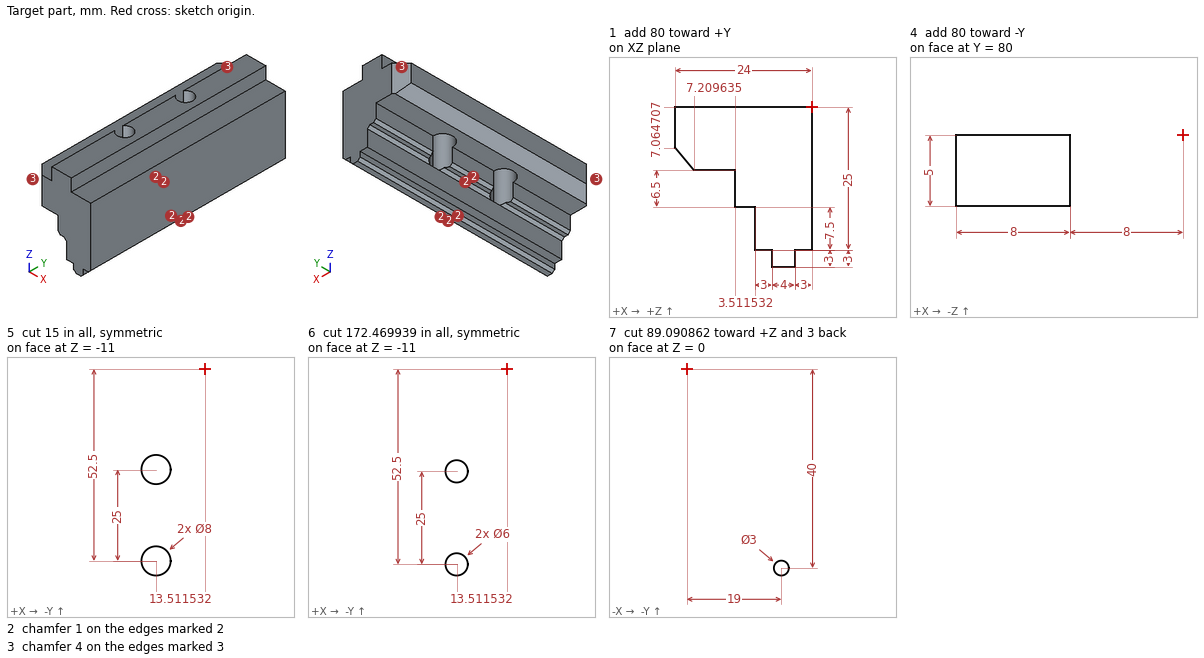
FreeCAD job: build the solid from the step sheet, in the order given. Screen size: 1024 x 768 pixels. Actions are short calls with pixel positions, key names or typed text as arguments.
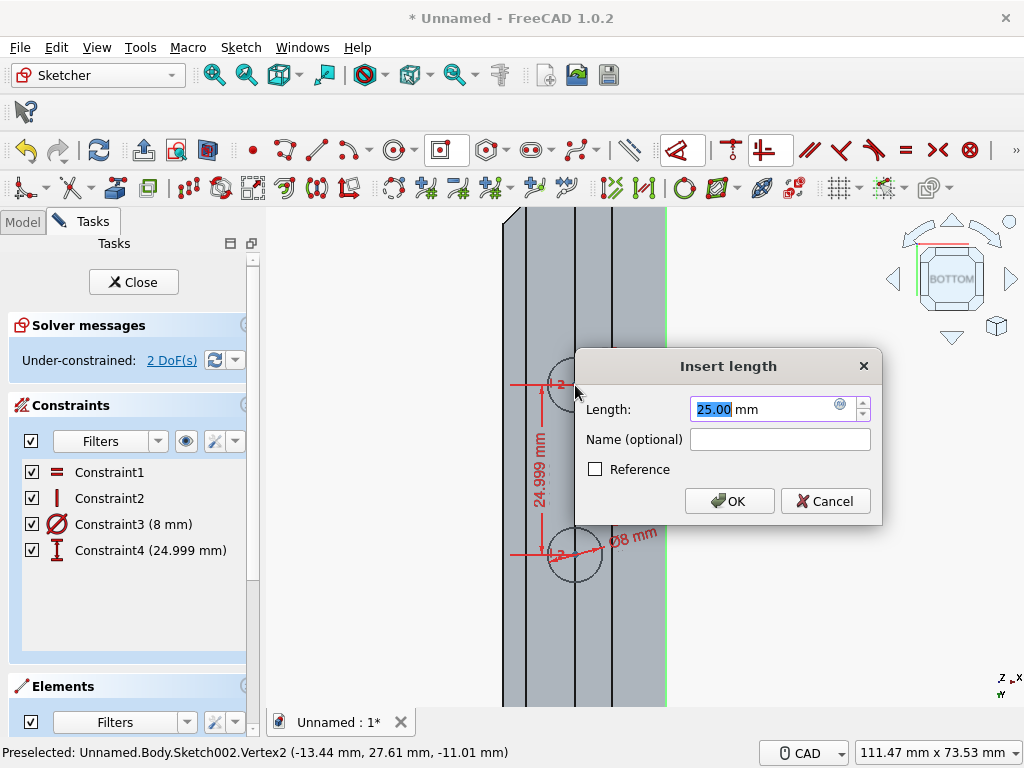
text(25)
key(Return)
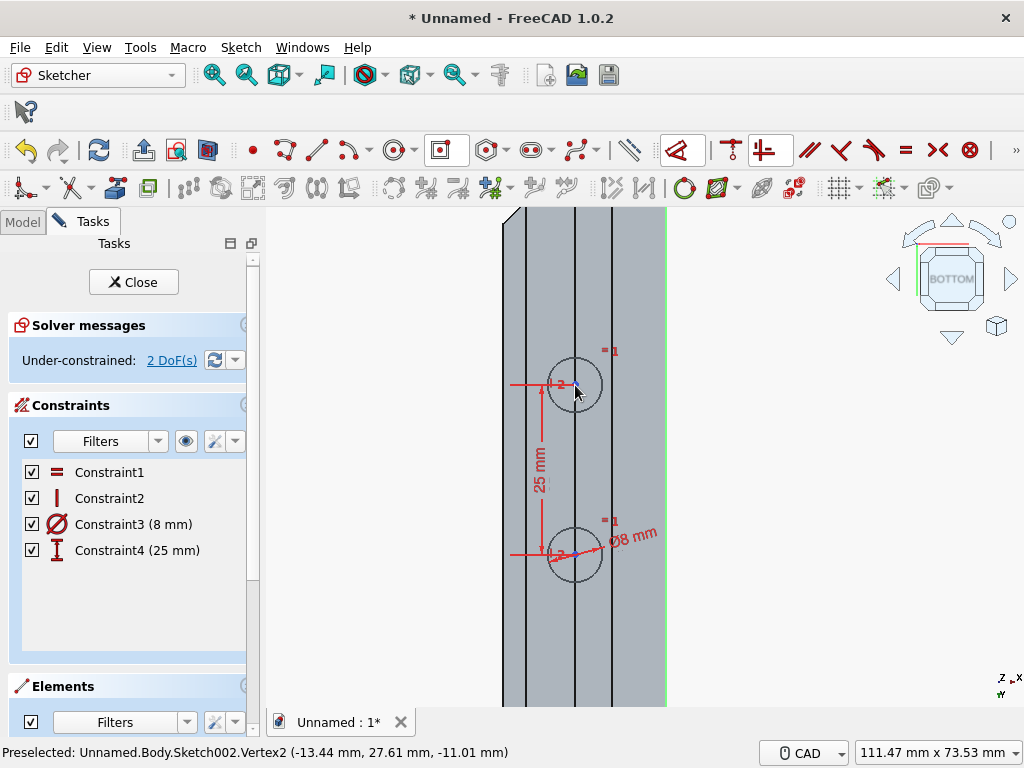
click(575, 555)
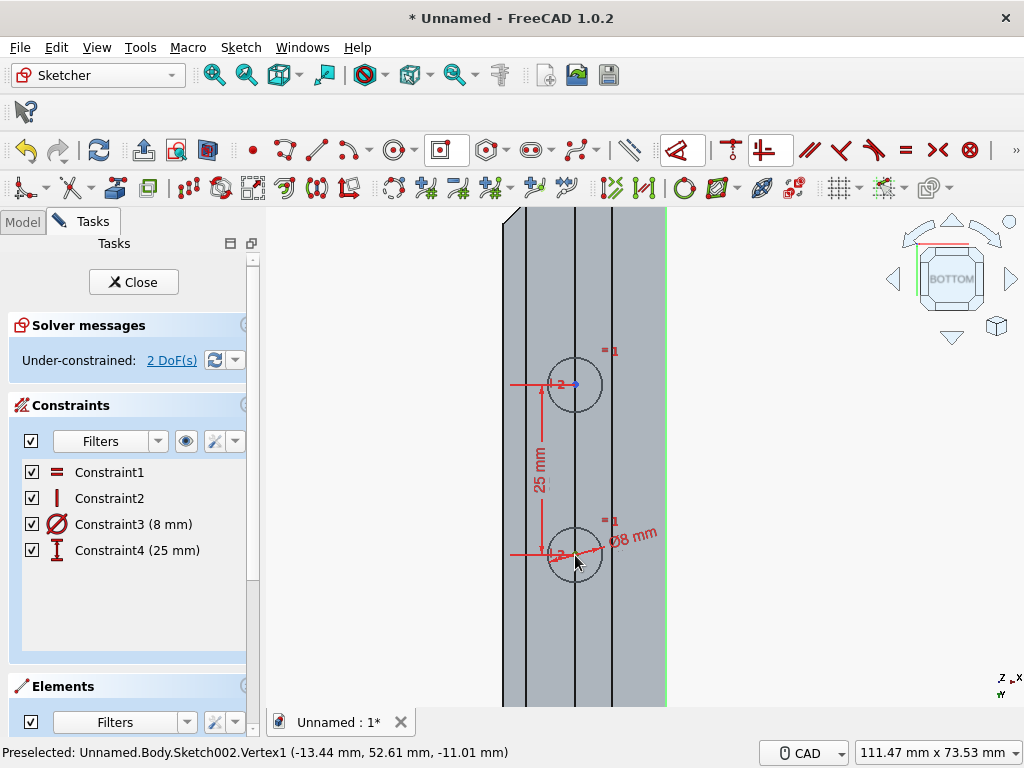
click(700, 150)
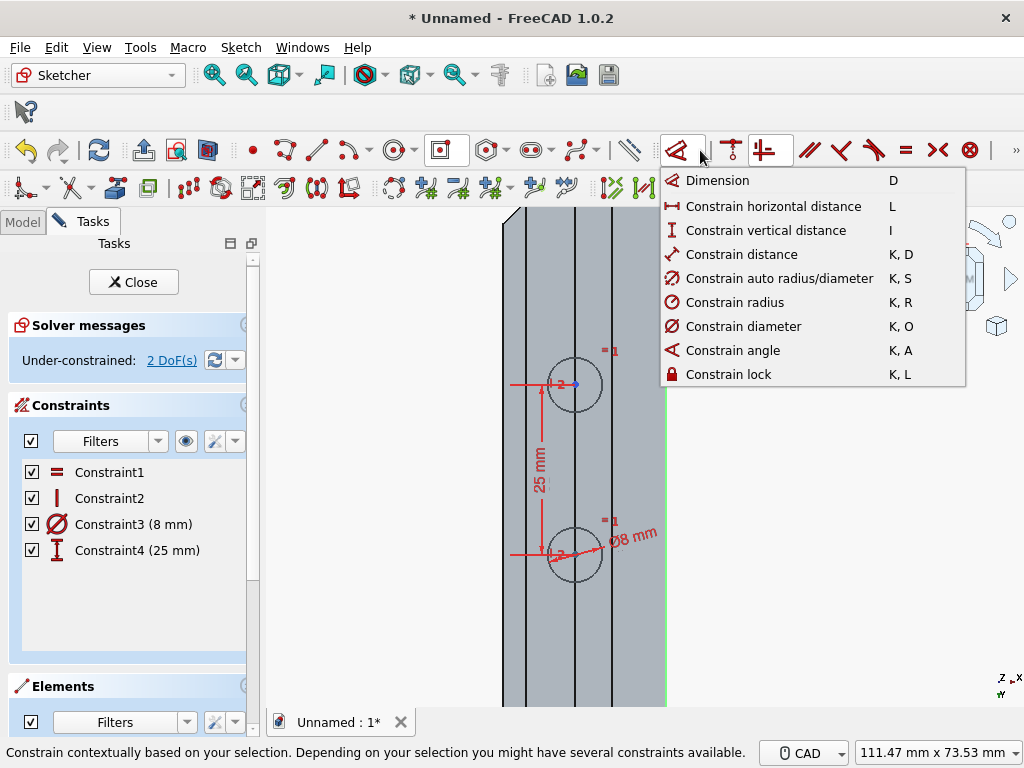
click(813, 230)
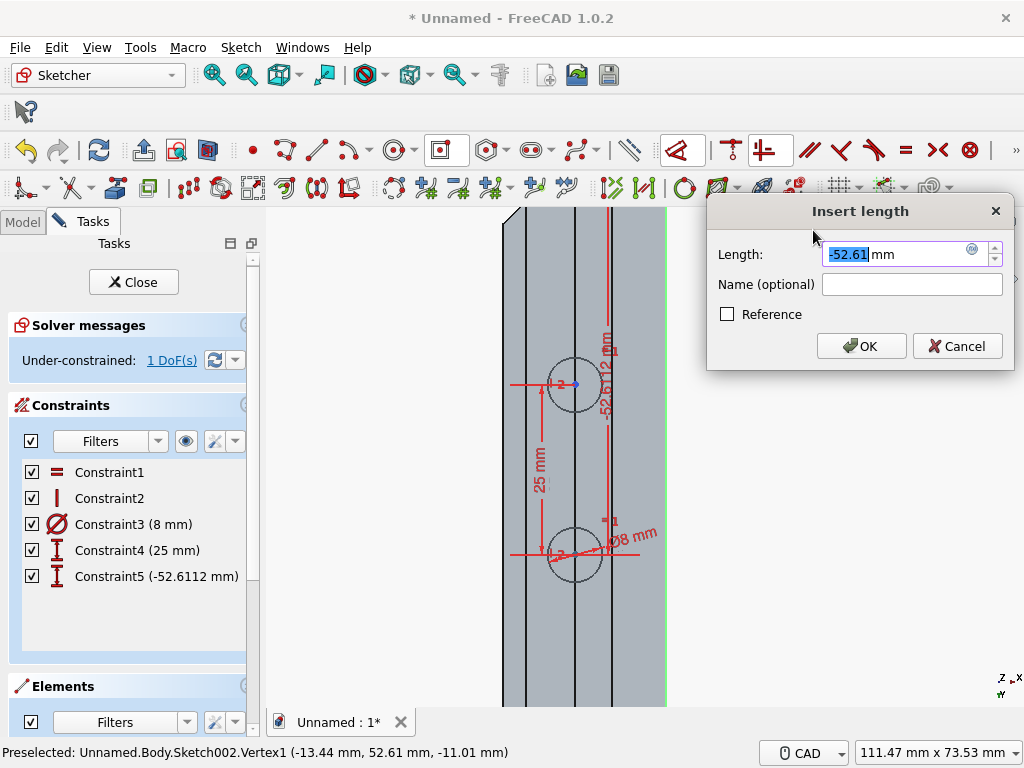
text(-52.5)
key(Return)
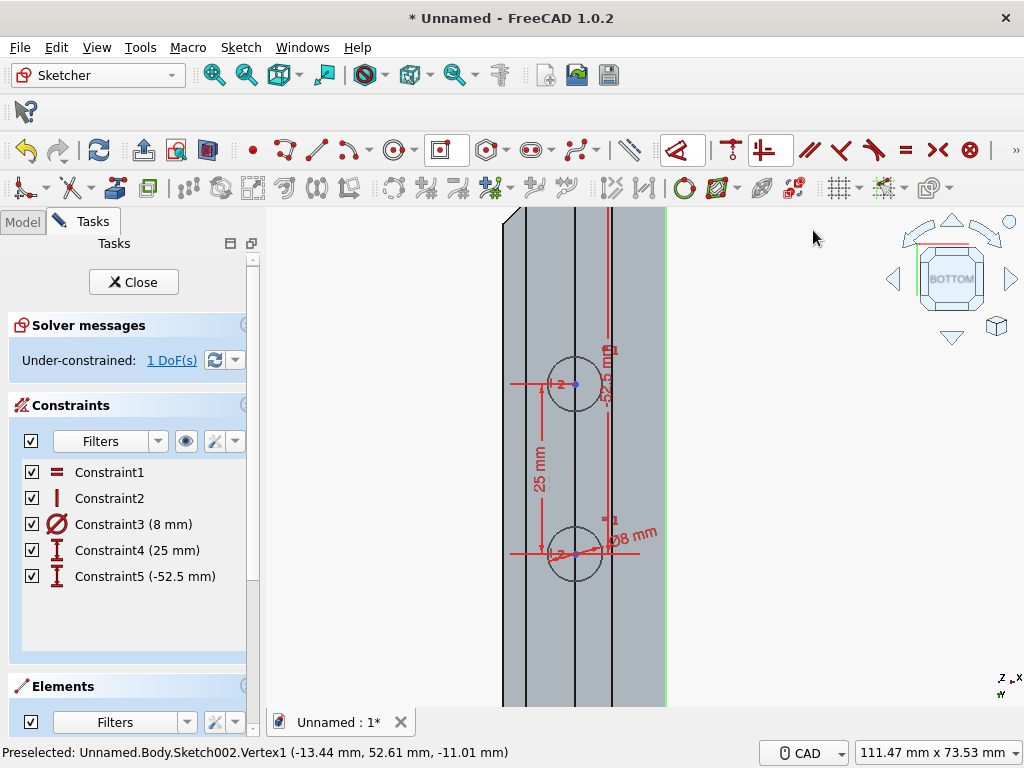
click(575, 554)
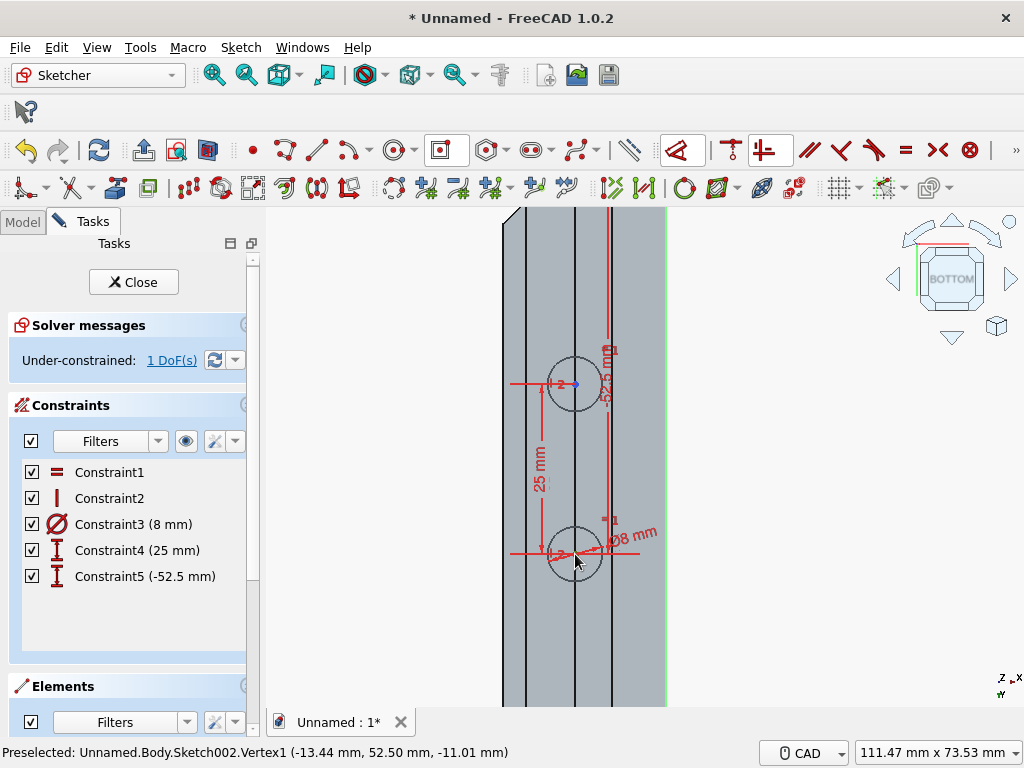
key(l)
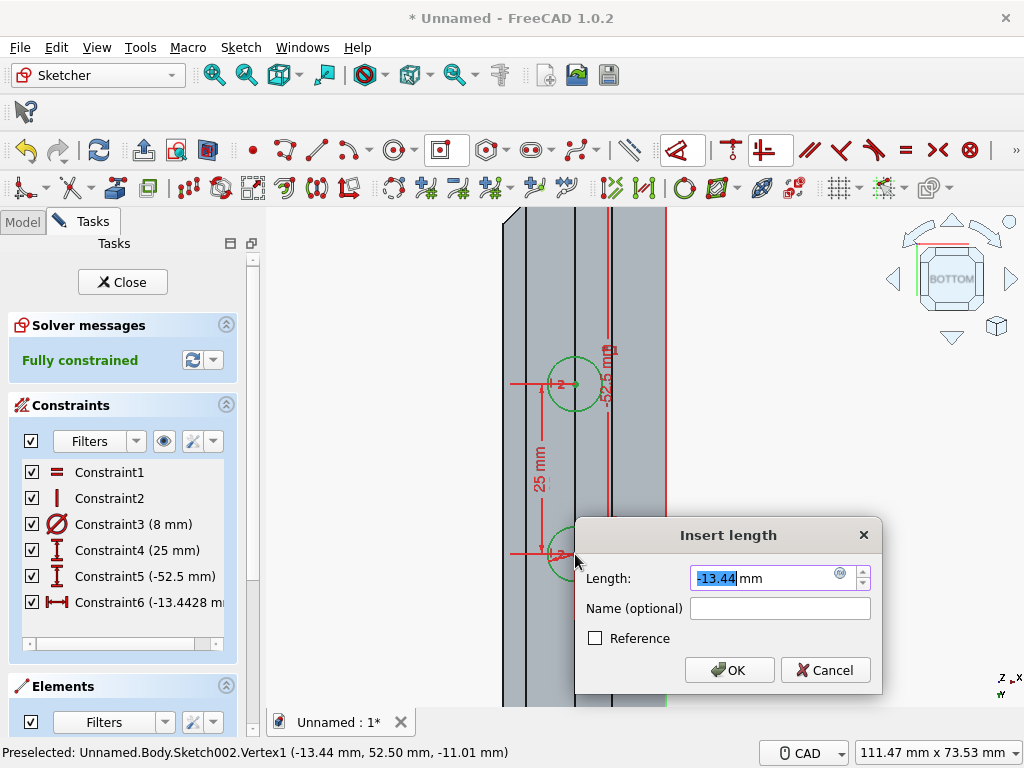
text(-13.511532)
key(Return)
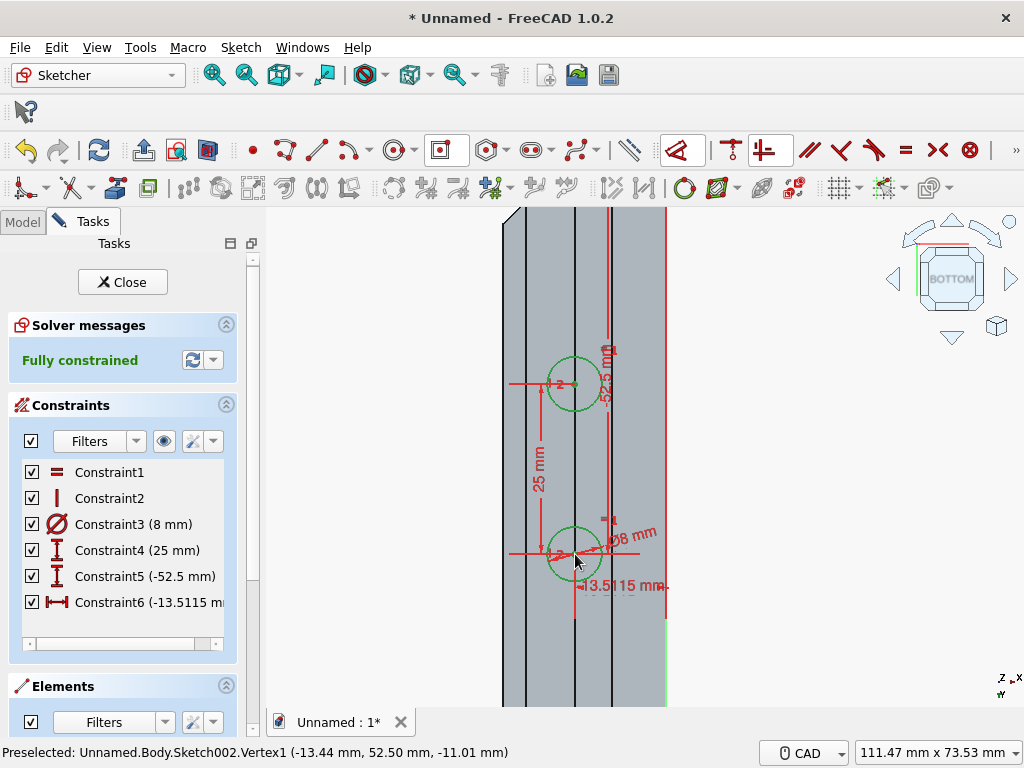
click(123, 282)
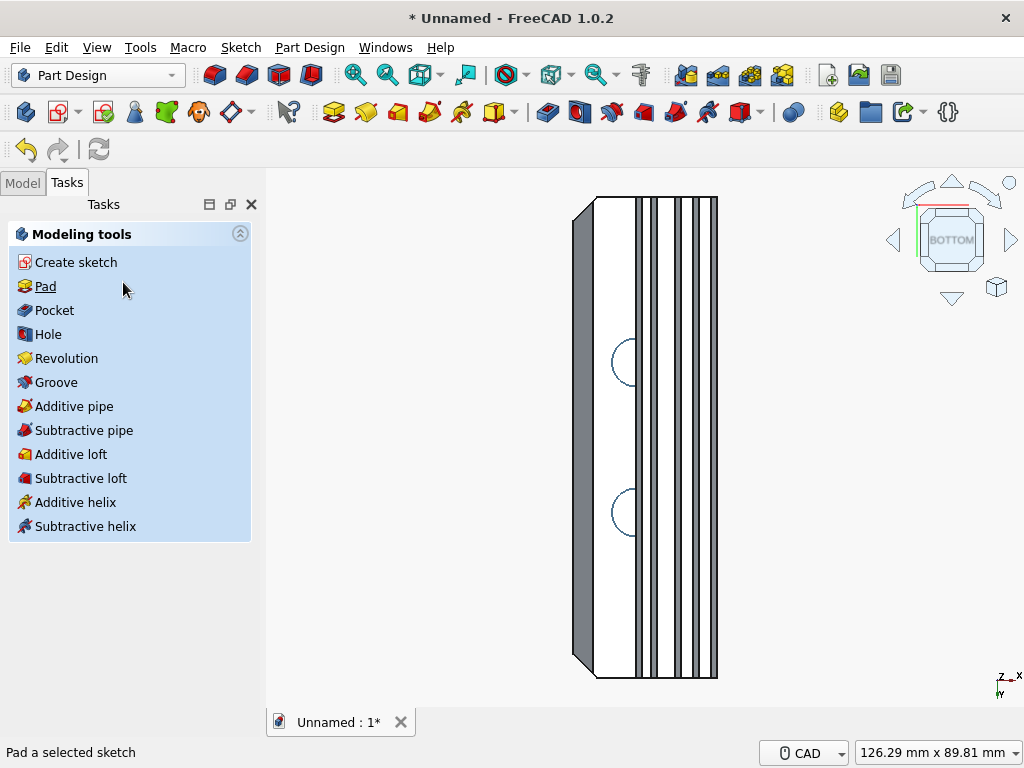
click(548, 112)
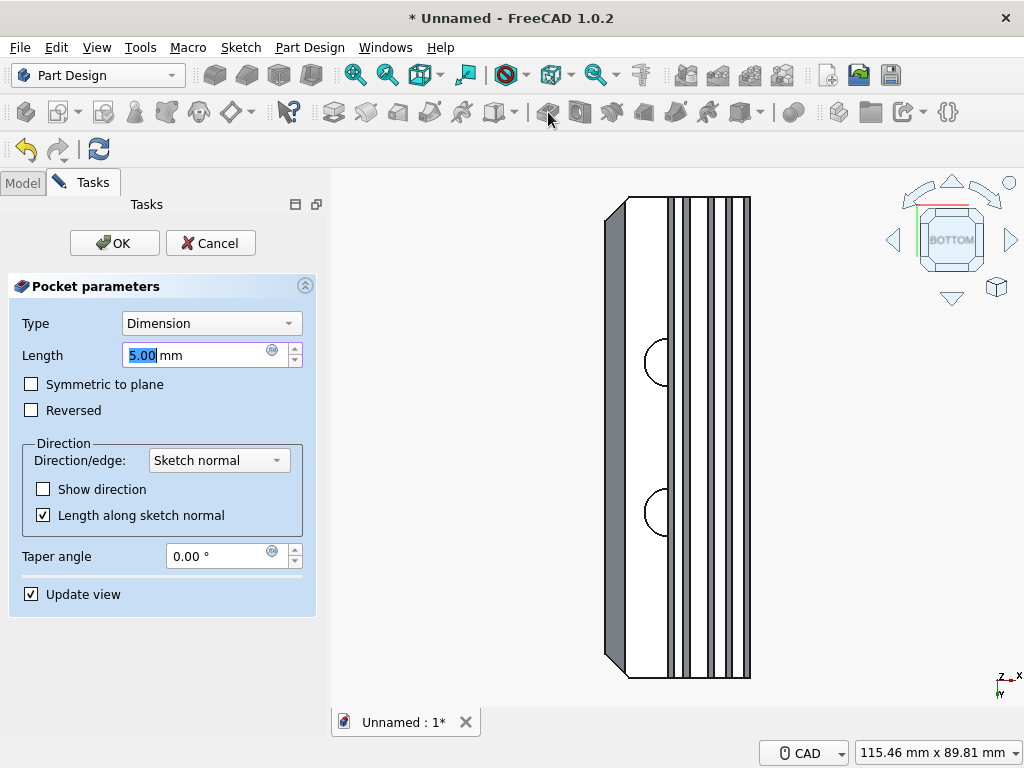
text(15)
key(Tab)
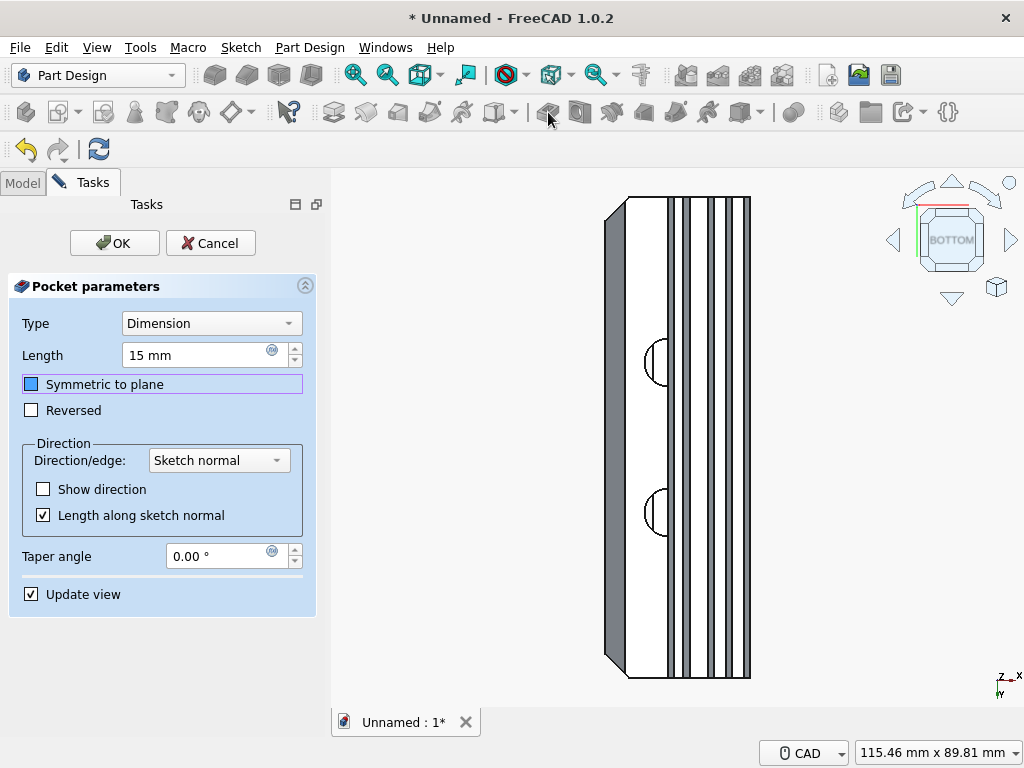
click(30, 384)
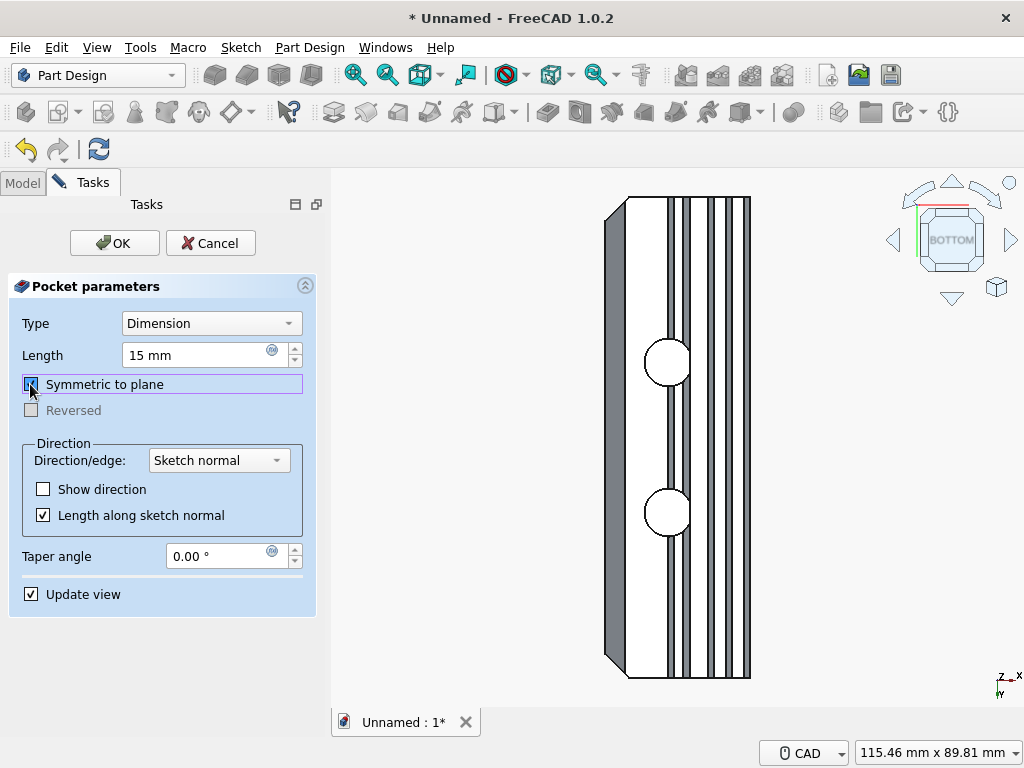
click(115, 243)